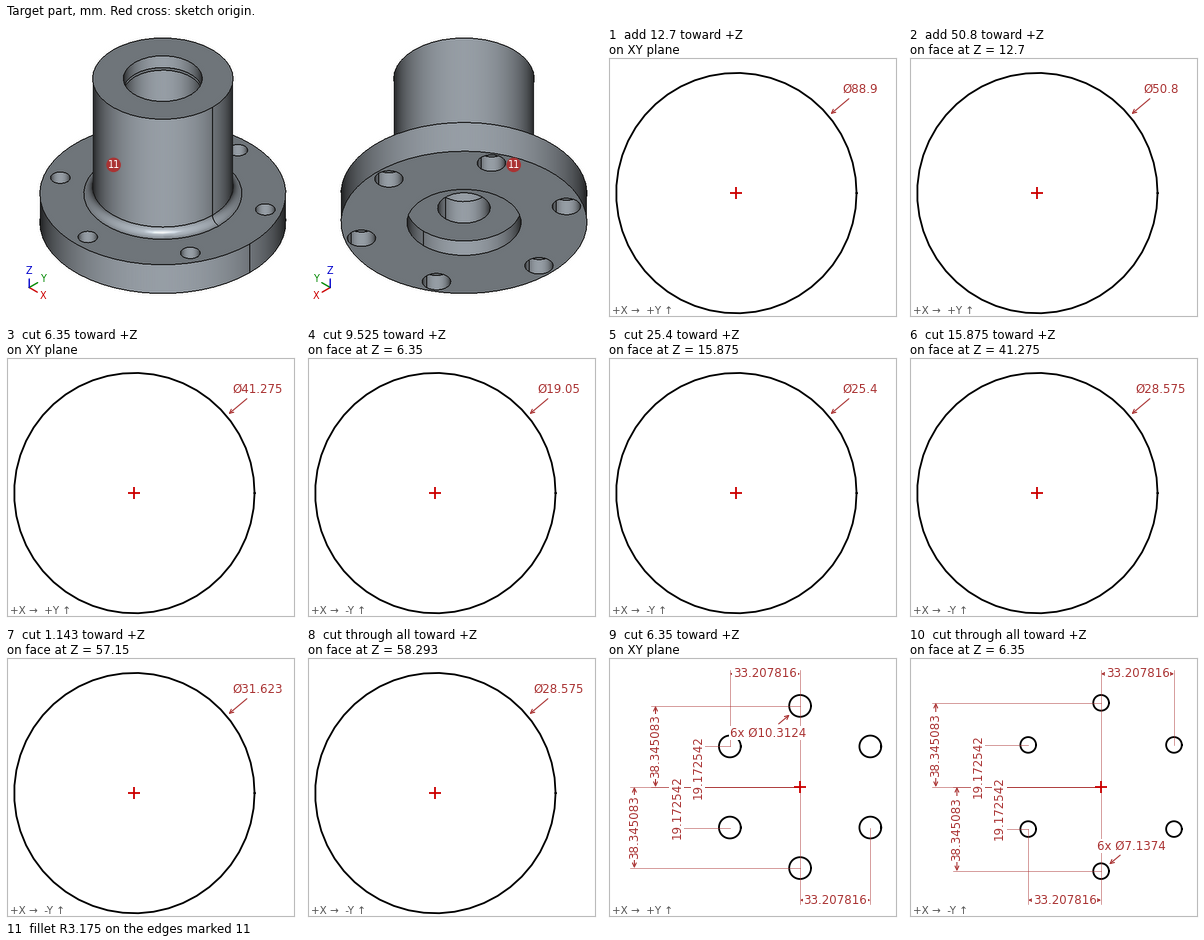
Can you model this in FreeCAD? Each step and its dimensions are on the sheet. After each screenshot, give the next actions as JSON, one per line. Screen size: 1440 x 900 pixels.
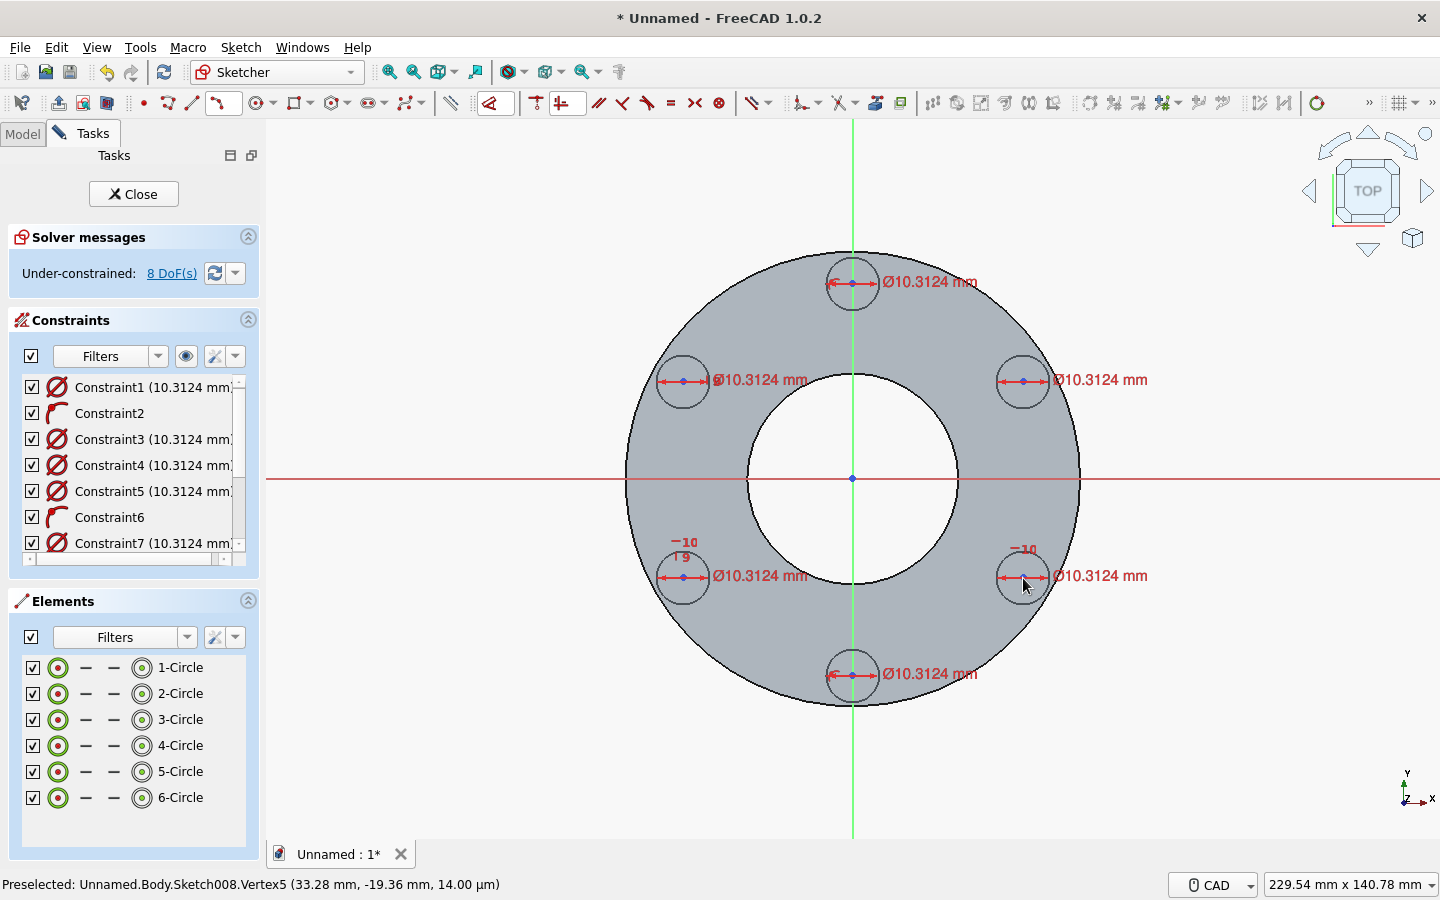
{"action": "left_click", "coordinate": [1023, 578]}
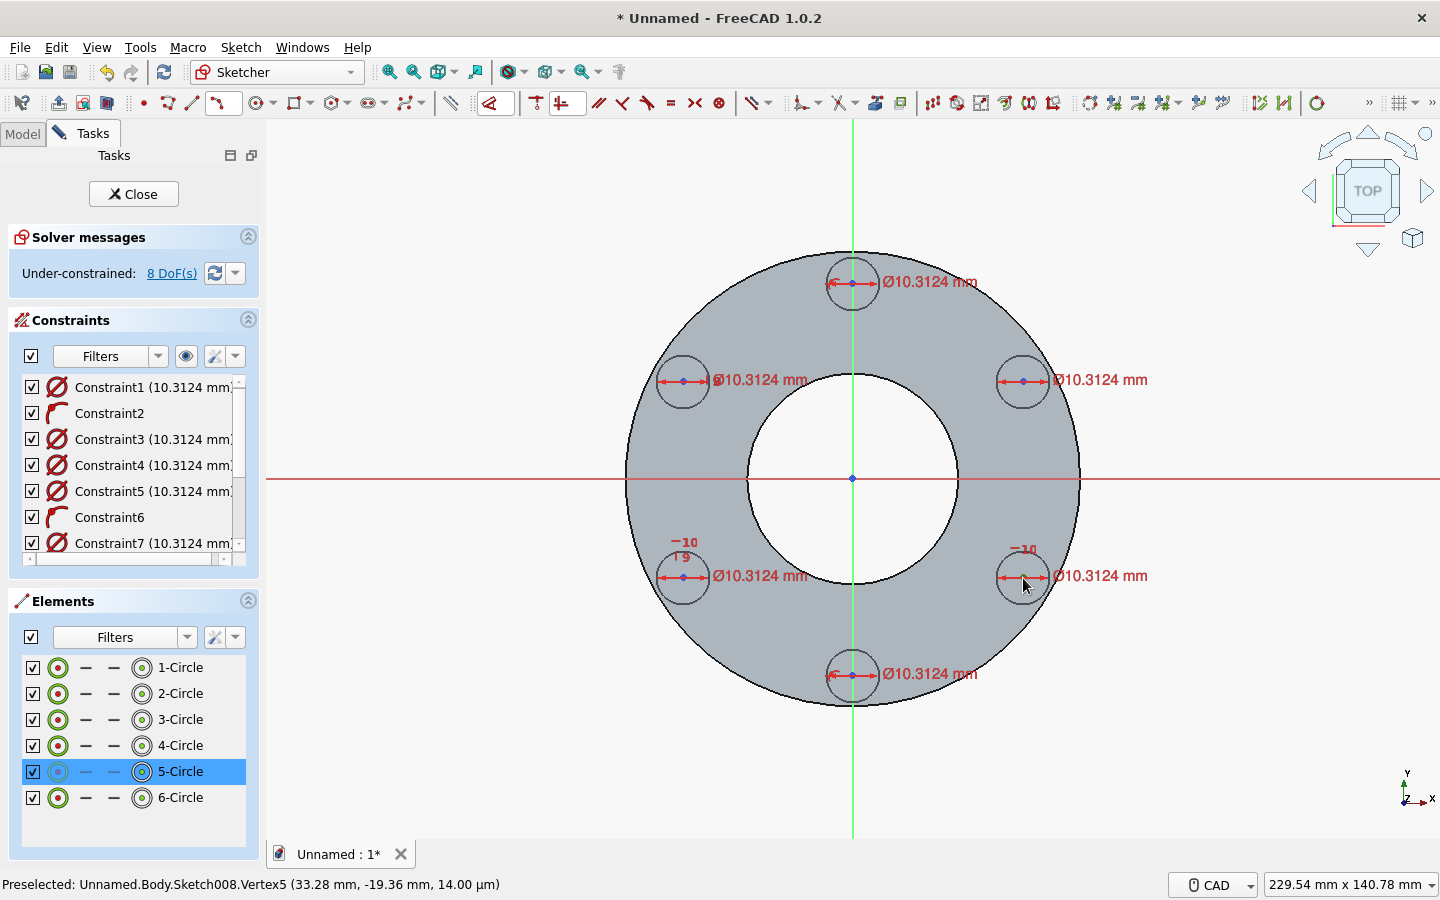
{"action": "left_click", "coordinate": [1023, 382]}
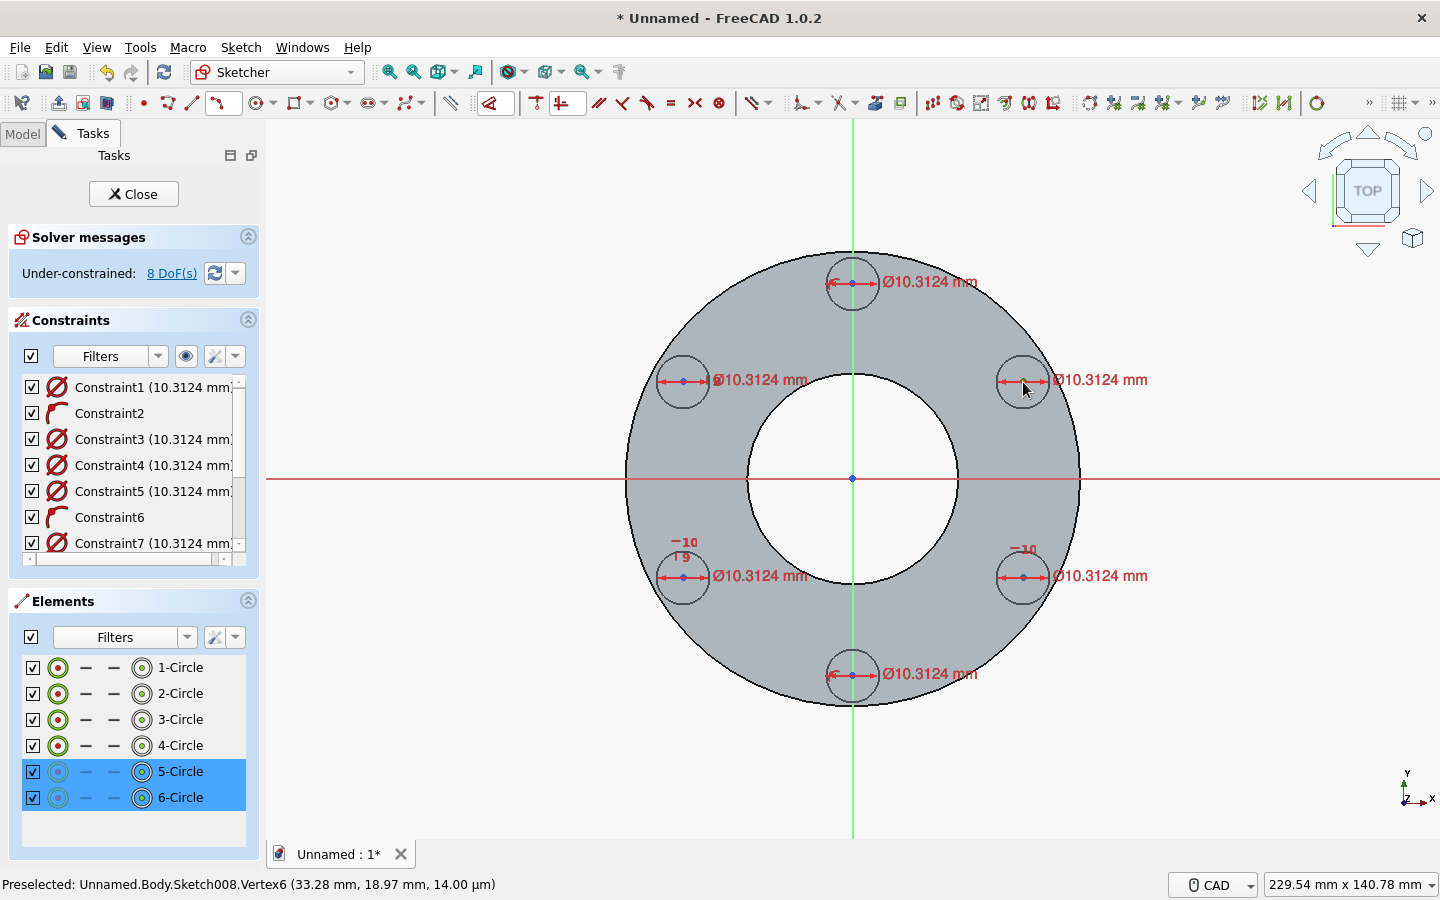
{"action": "left_click", "coordinate": [580, 104]}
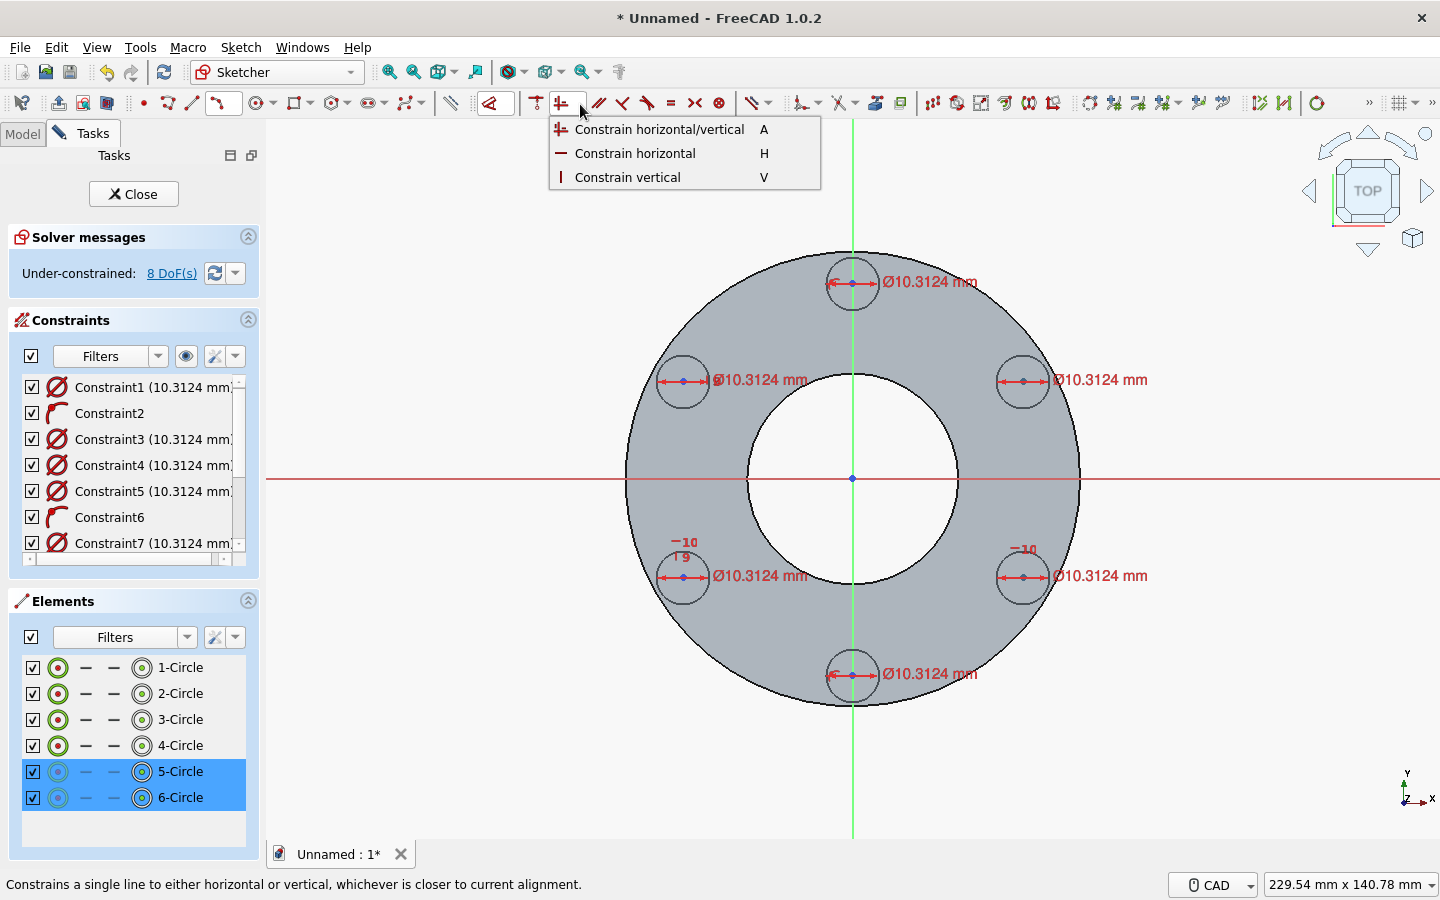
{"action": "left_click", "coordinate": [685, 177]}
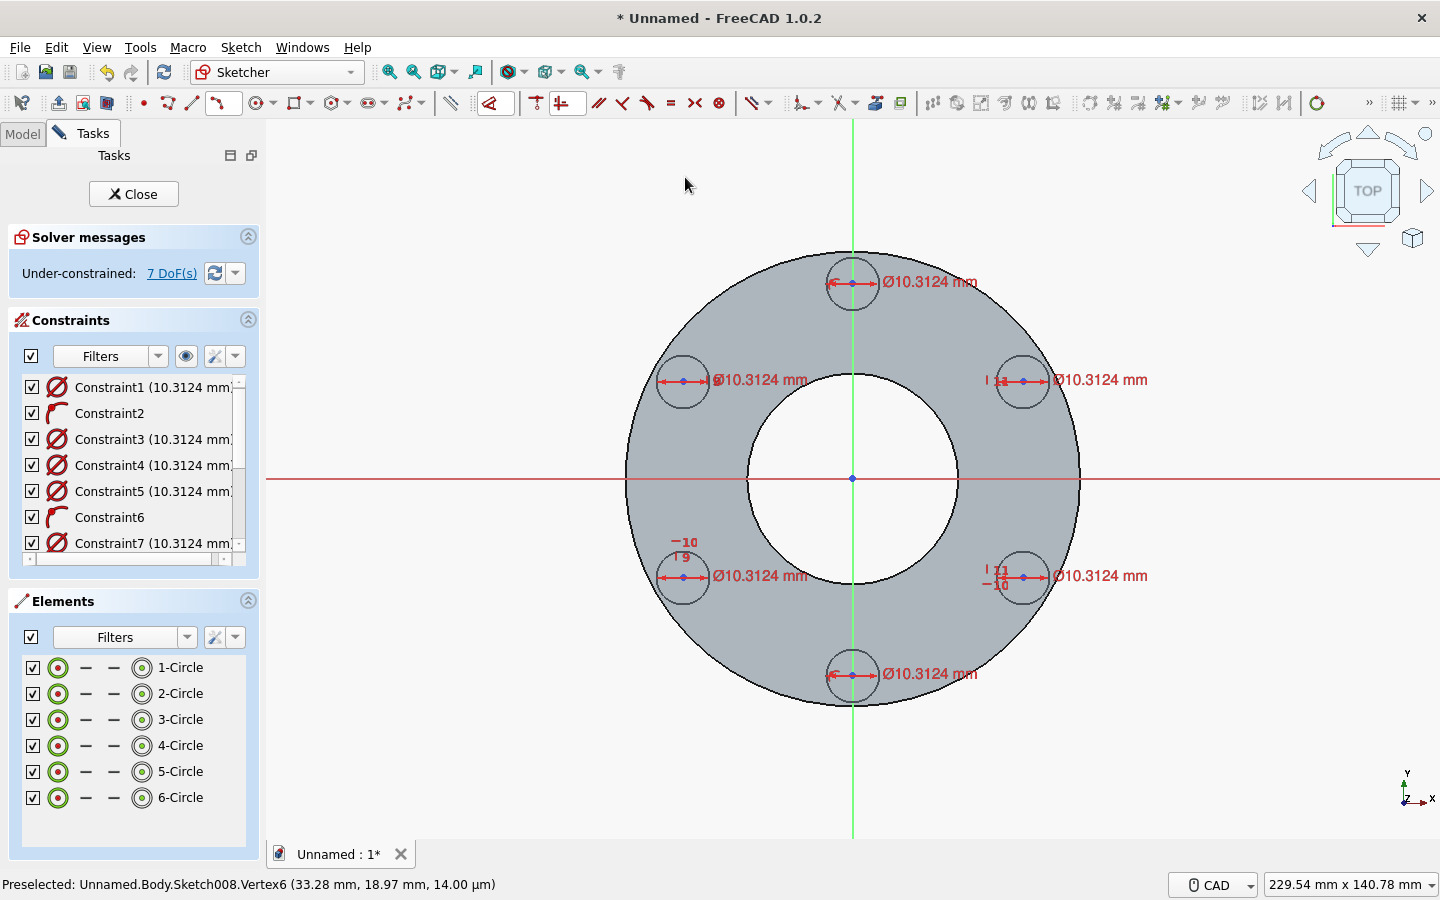
{"action": "left_click", "coordinate": [683, 382]}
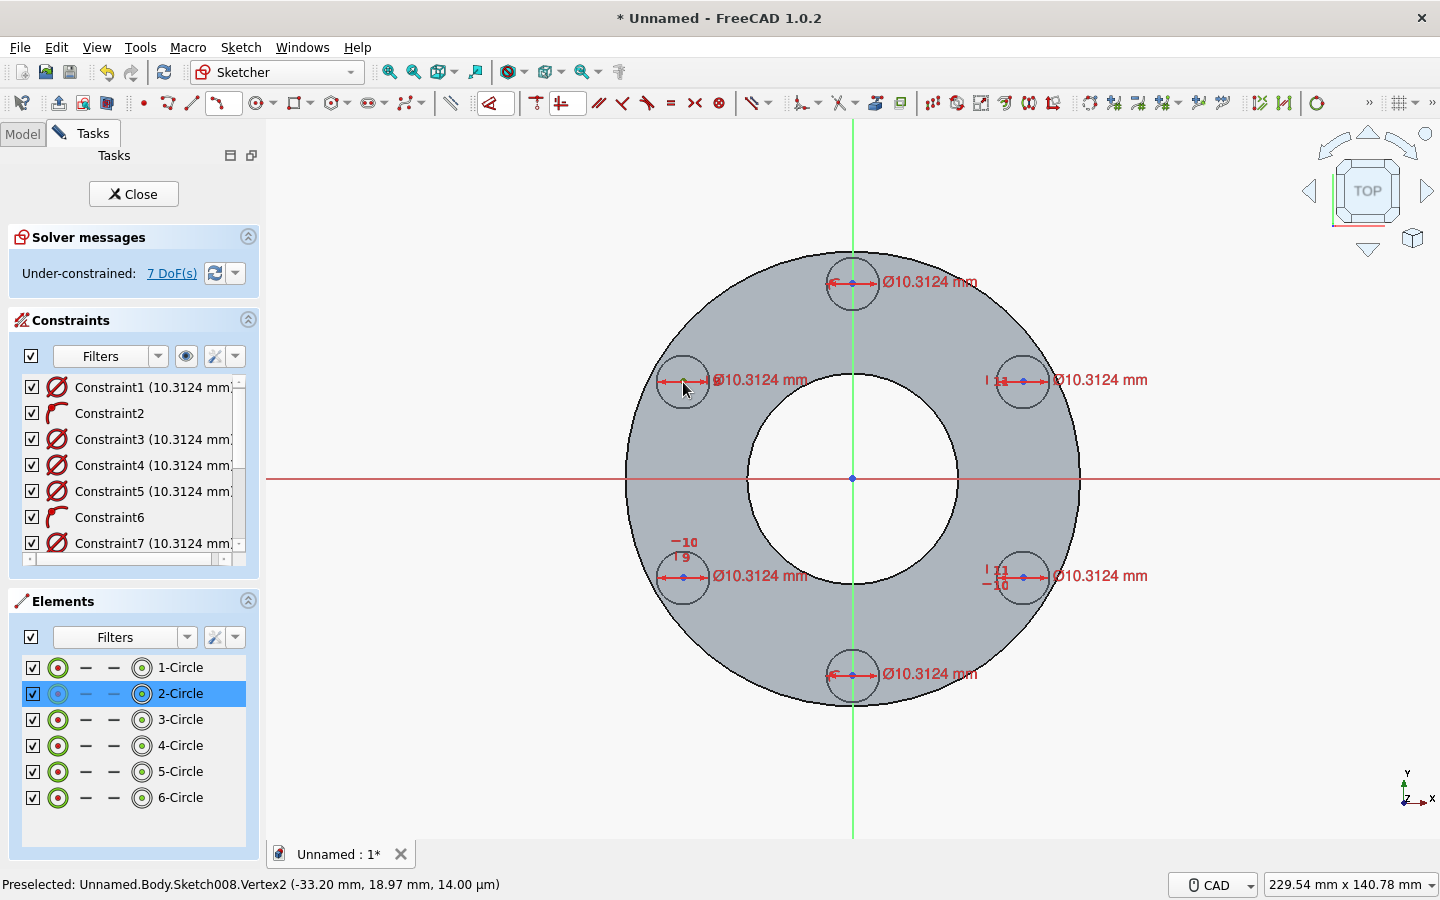
{"action": "left_click", "coordinate": [1023, 382]}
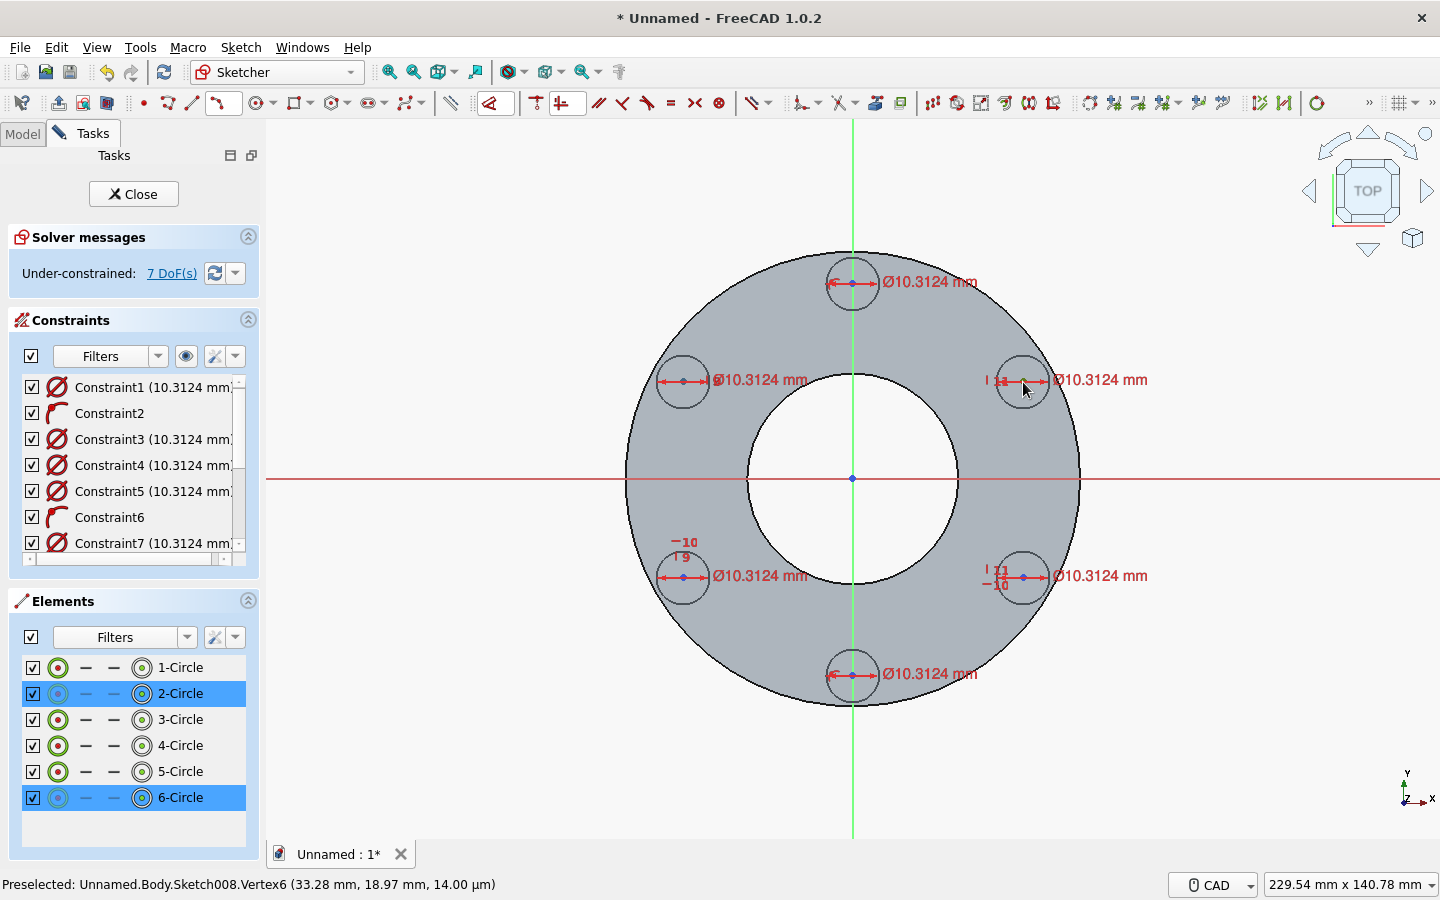
{"action": "key", "text": "h"}